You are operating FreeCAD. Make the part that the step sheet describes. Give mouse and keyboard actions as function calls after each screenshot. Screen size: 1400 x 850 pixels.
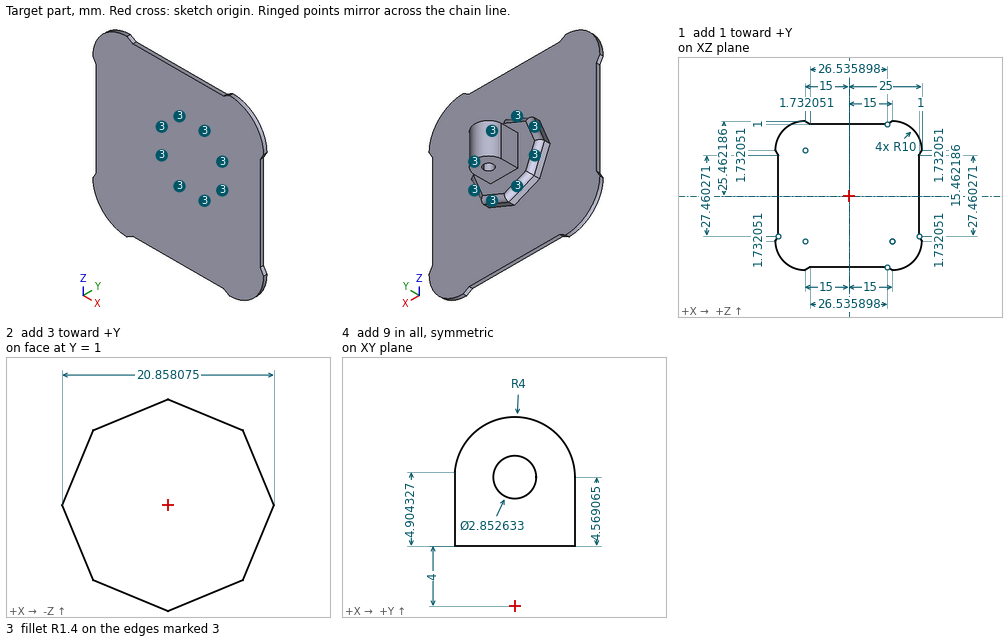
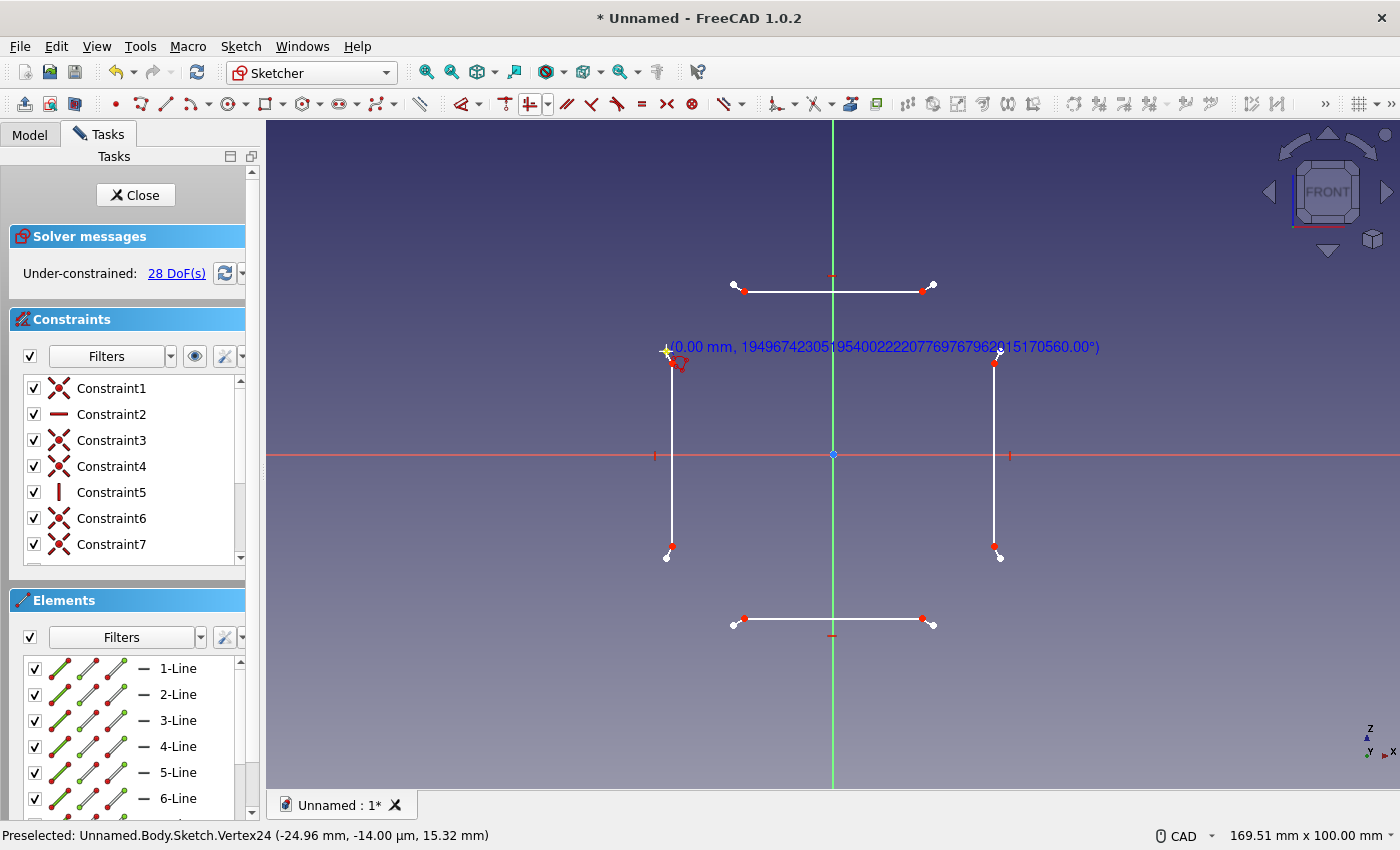
click(208, 104)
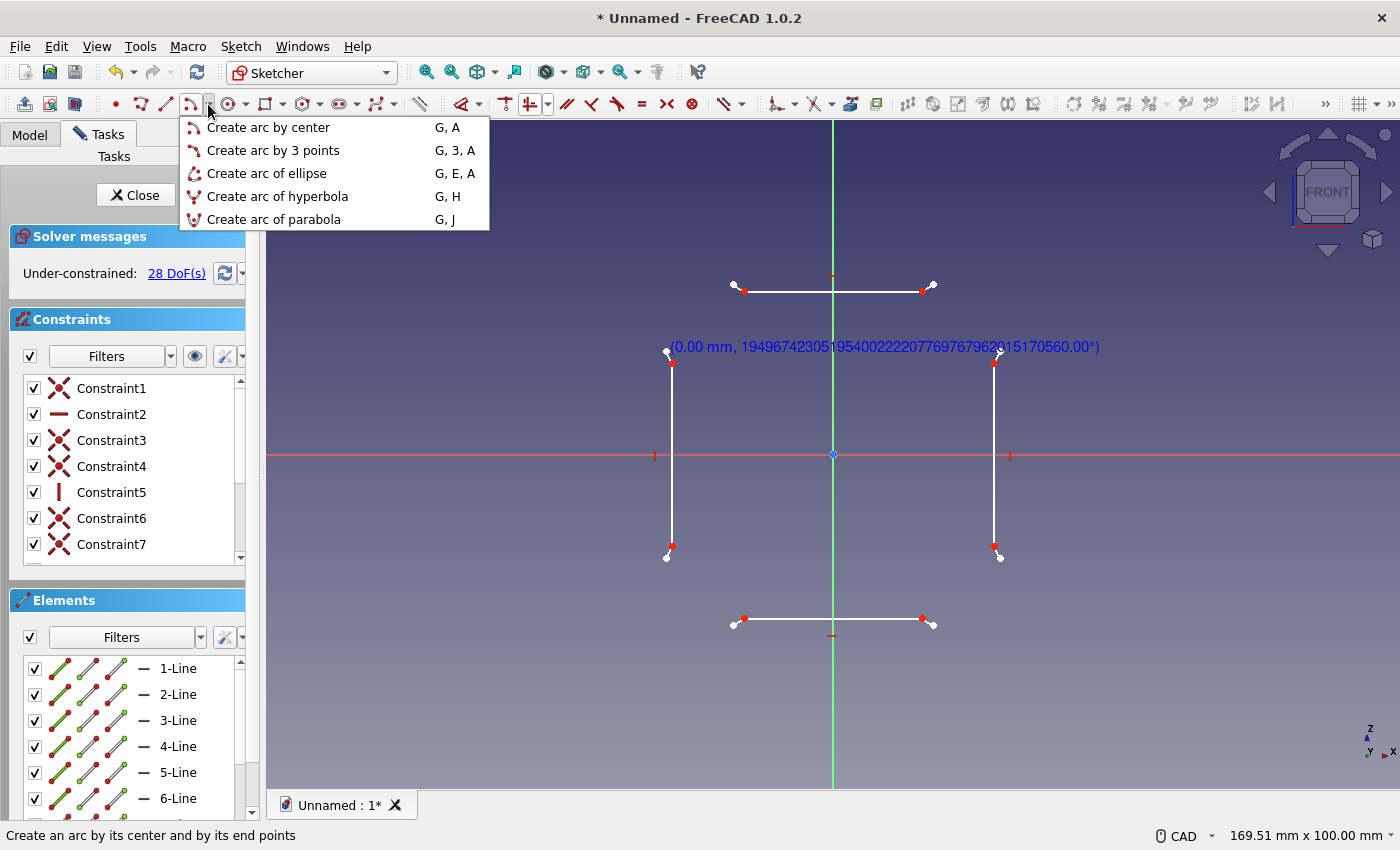
click(334, 150)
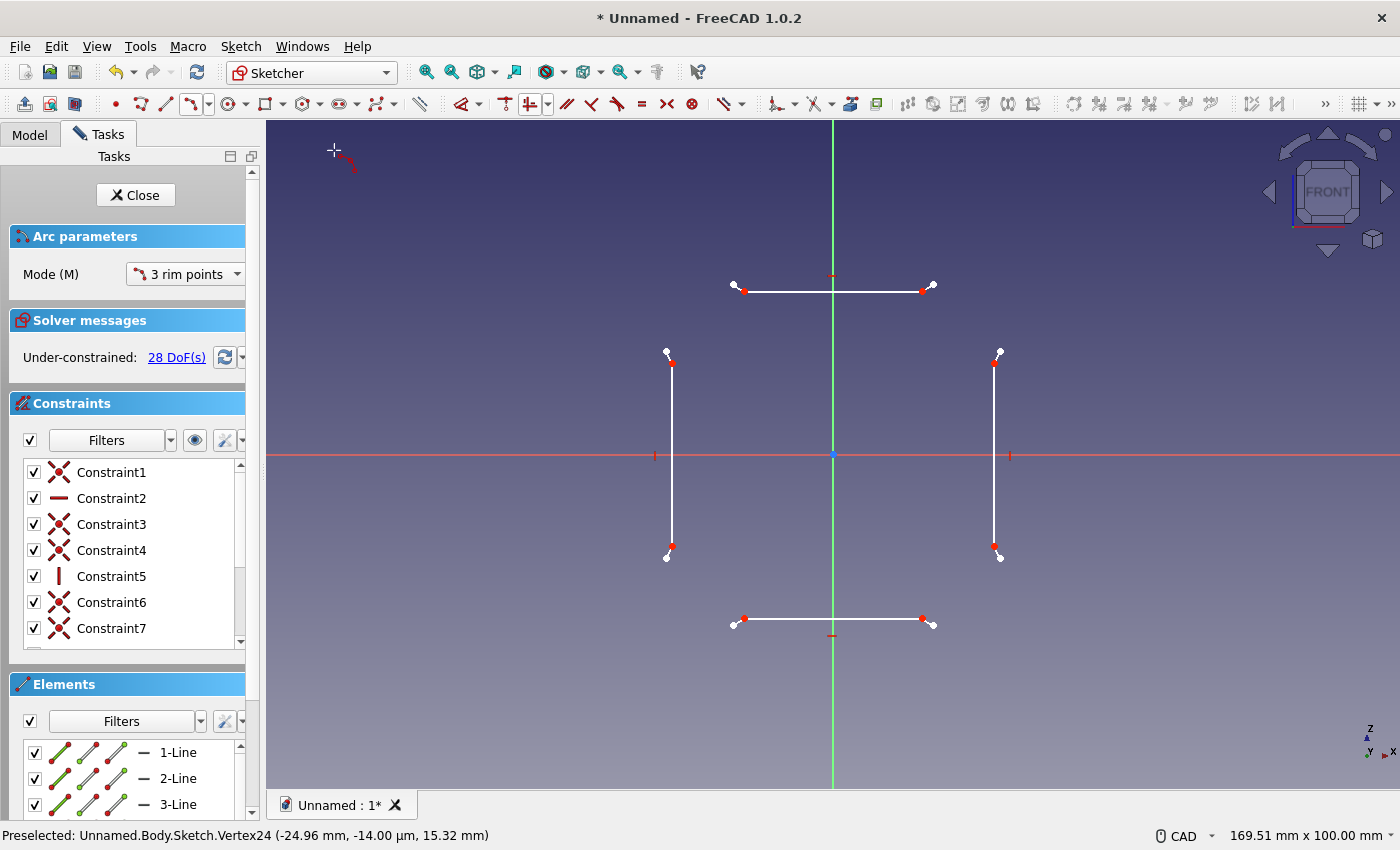
scroll(933, 284, up, 5)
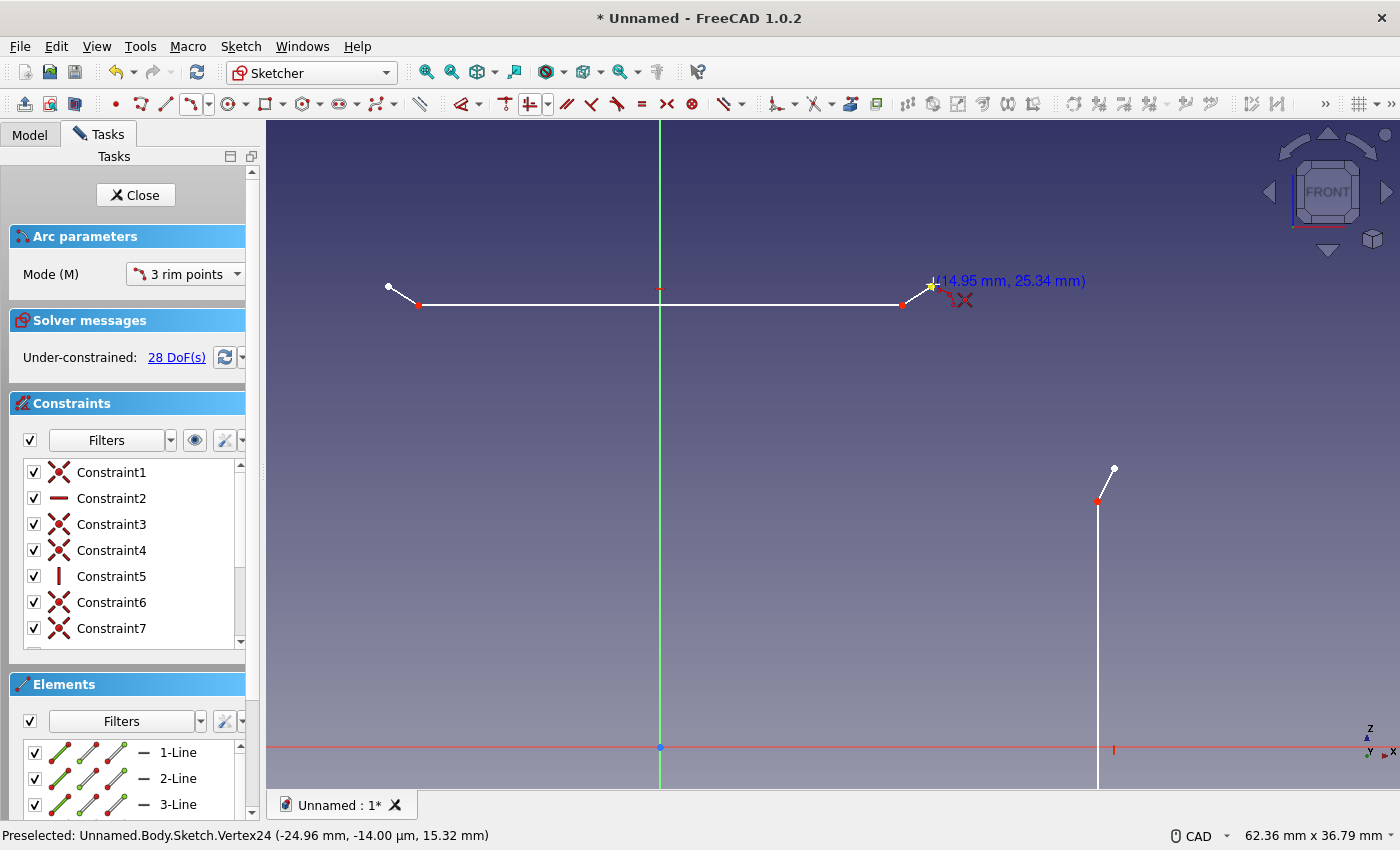
click(932, 286)
click(1114, 468)
click(1062, 337)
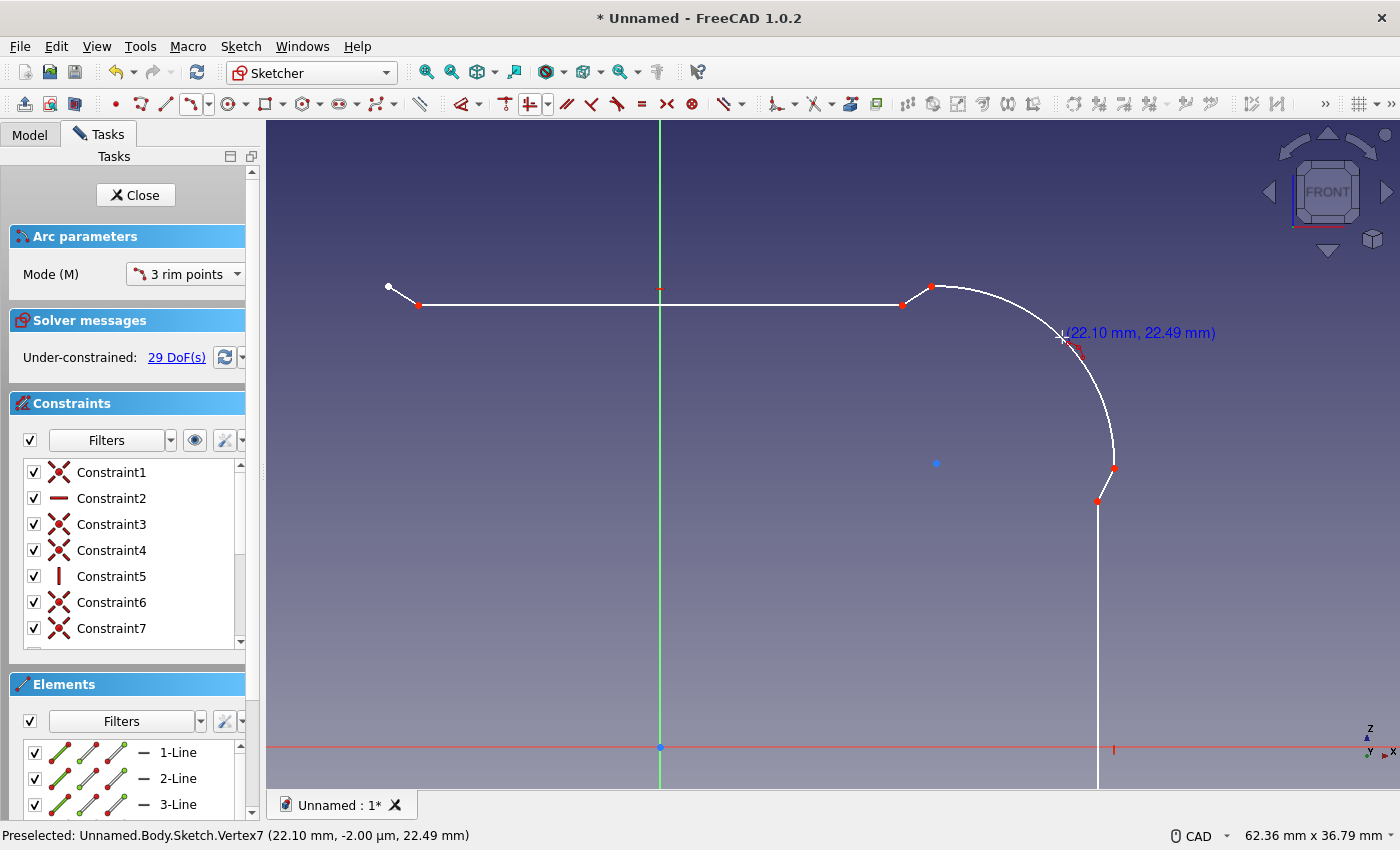
scroll(850, 216, down, 4)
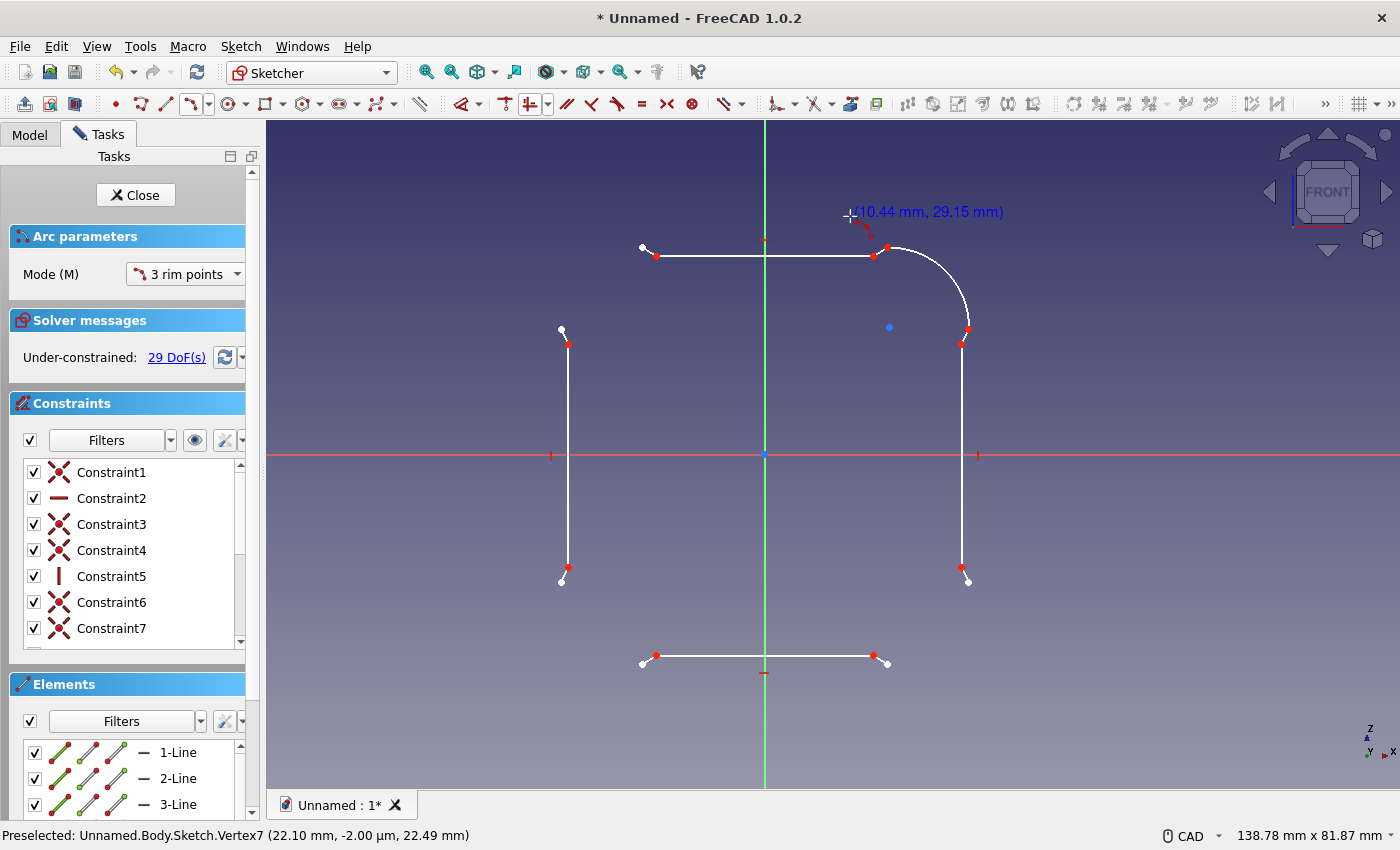
scroll(969, 581, up, 4)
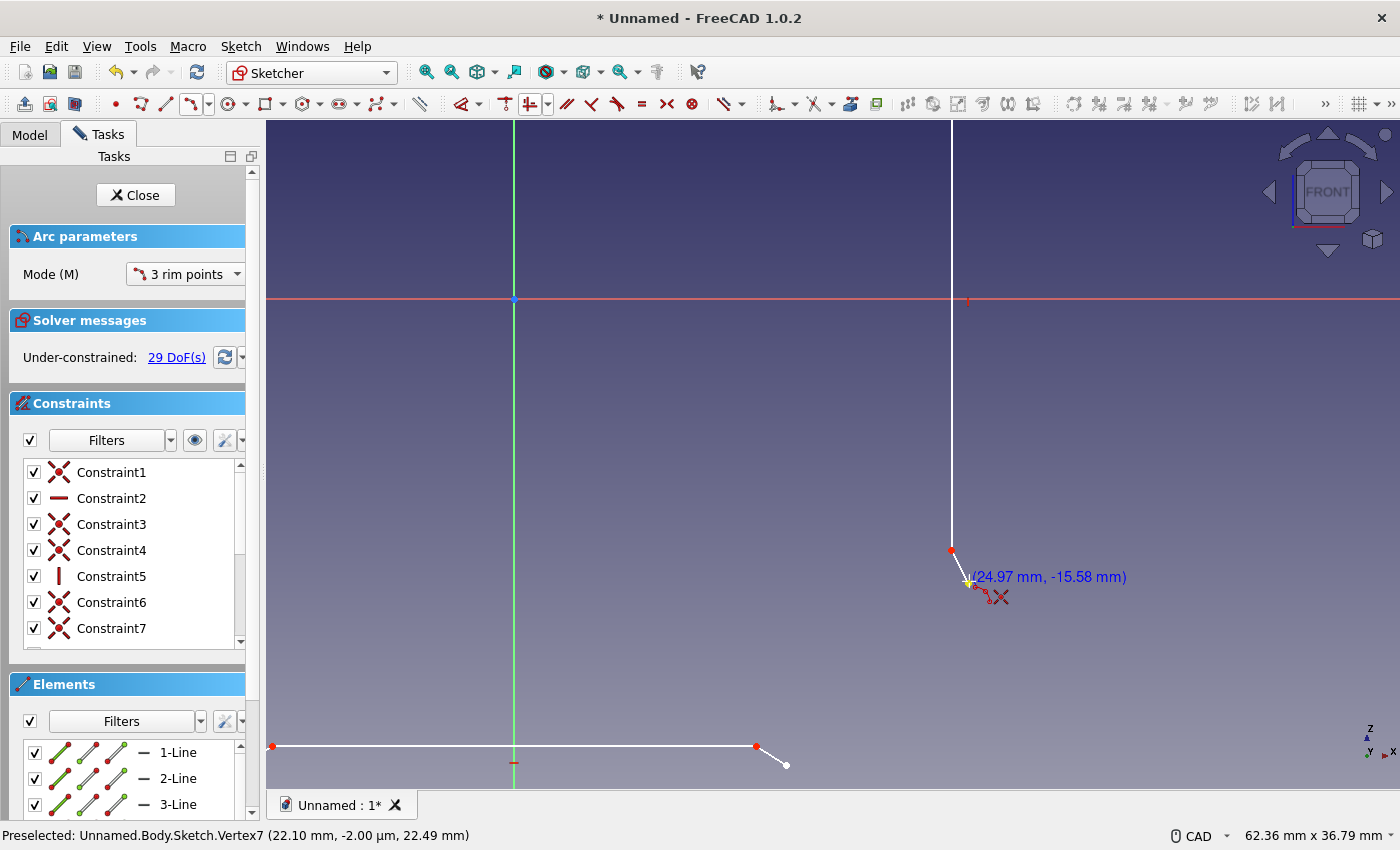
click(968, 583)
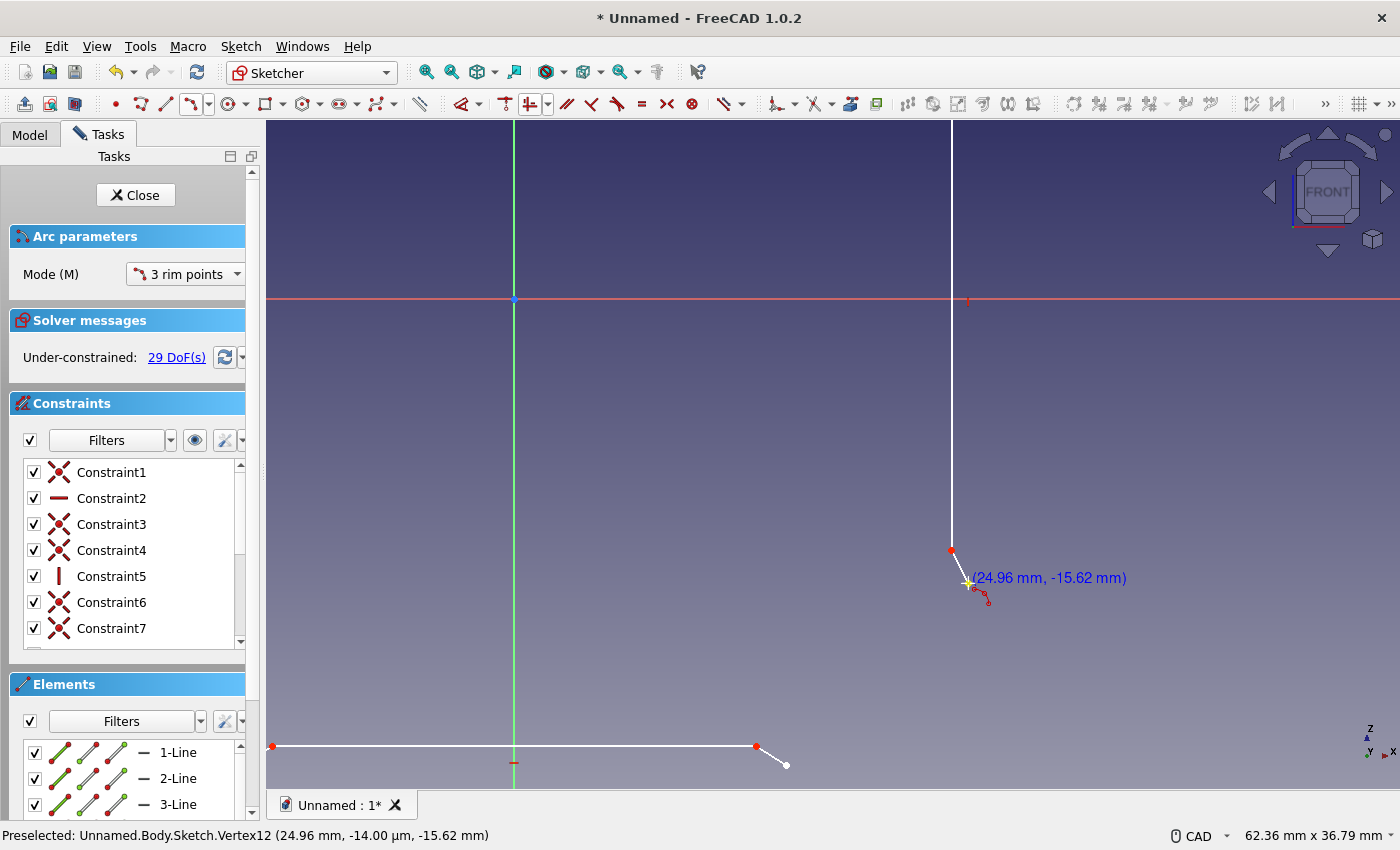
scroll(969, 581, down, 4)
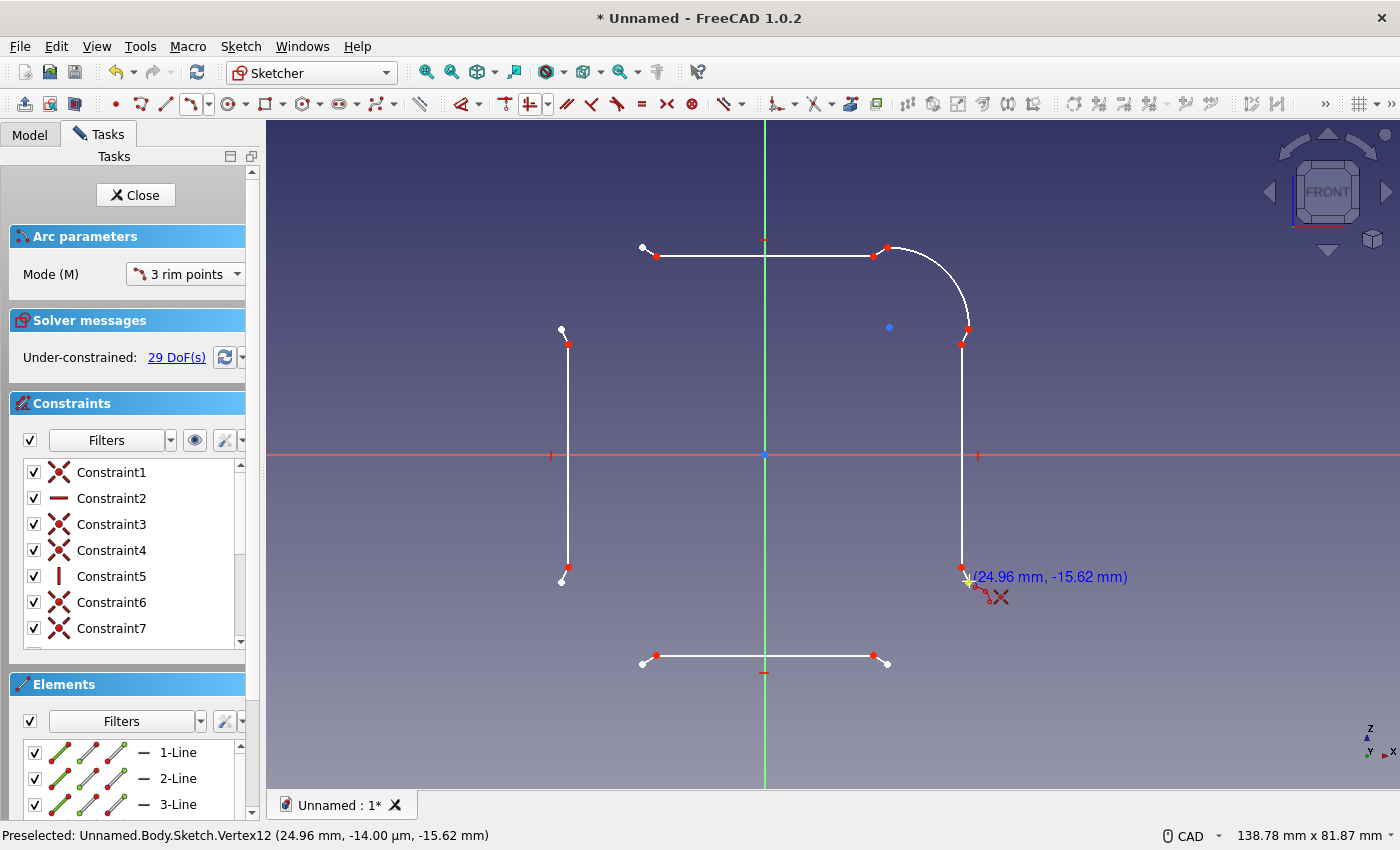
scroll(888, 663, up, 4)